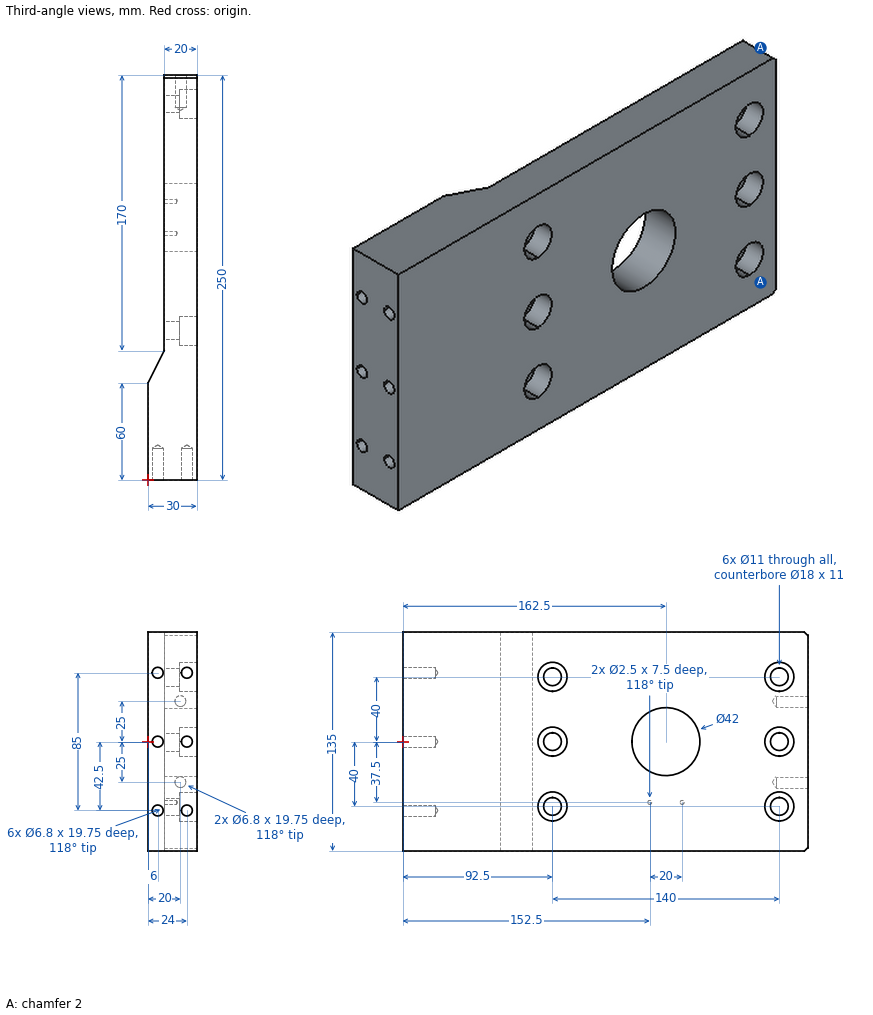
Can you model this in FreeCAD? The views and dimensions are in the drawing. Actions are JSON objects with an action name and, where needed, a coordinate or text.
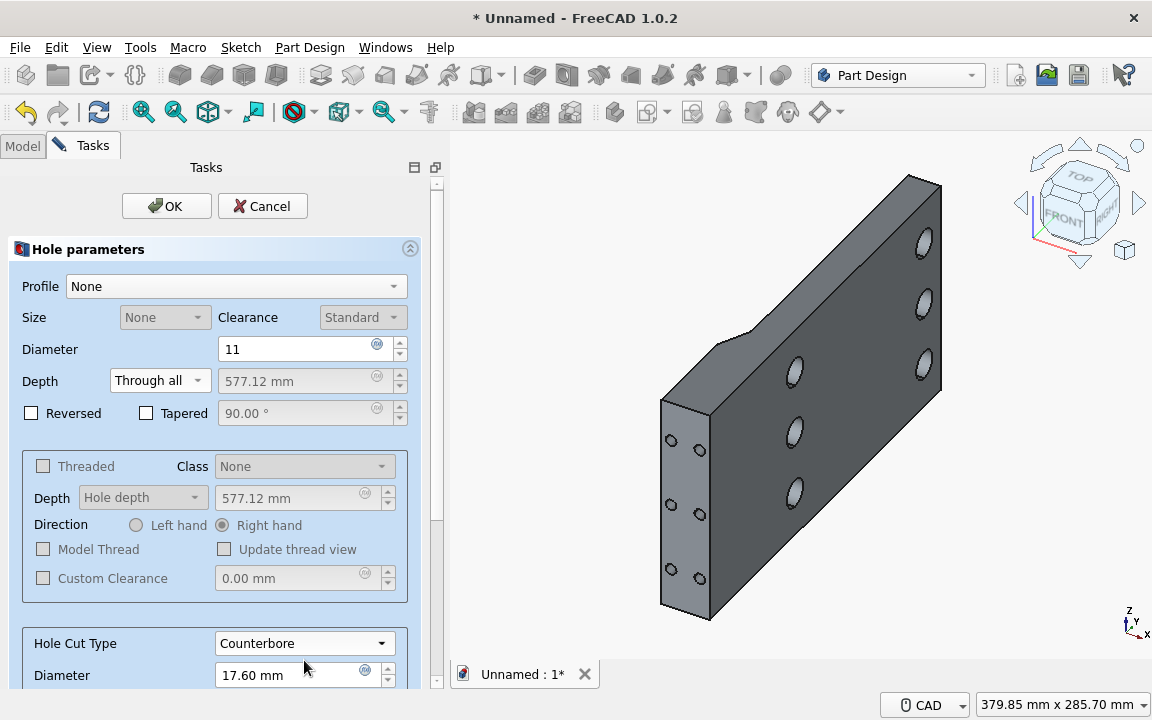
{"action": "triple_click", "coordinate": [298, 675]}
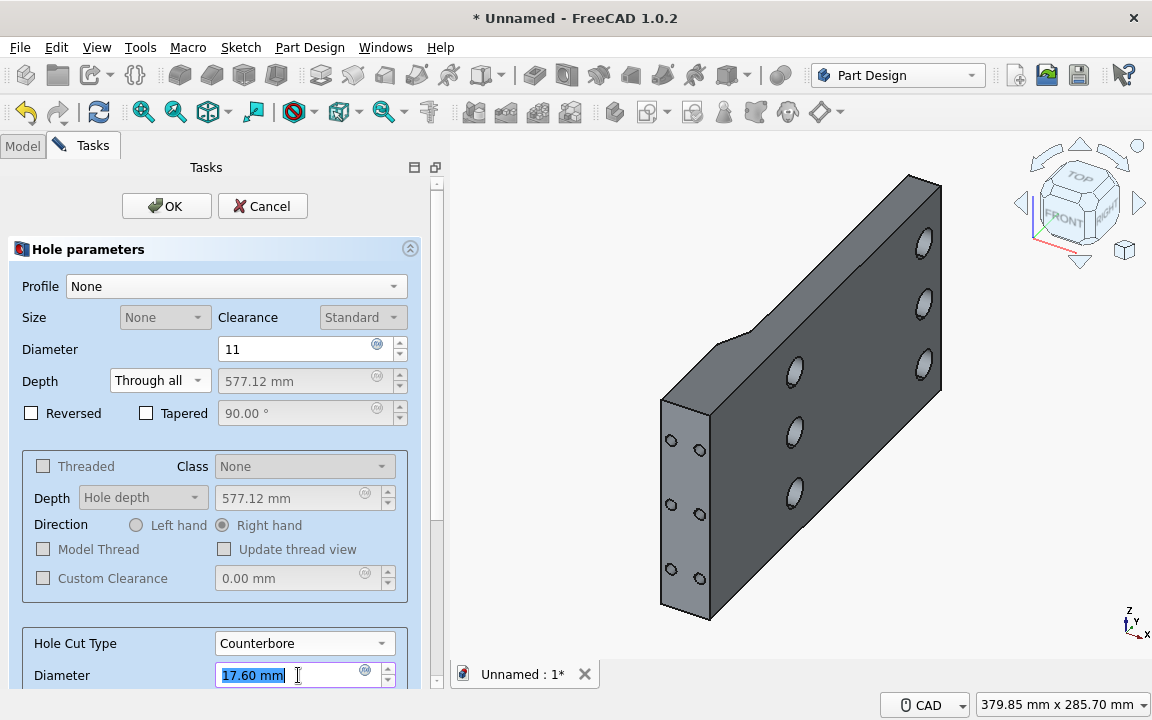
{"action": "type", "text": "18"}
{"action": "key", "text": "Tab"}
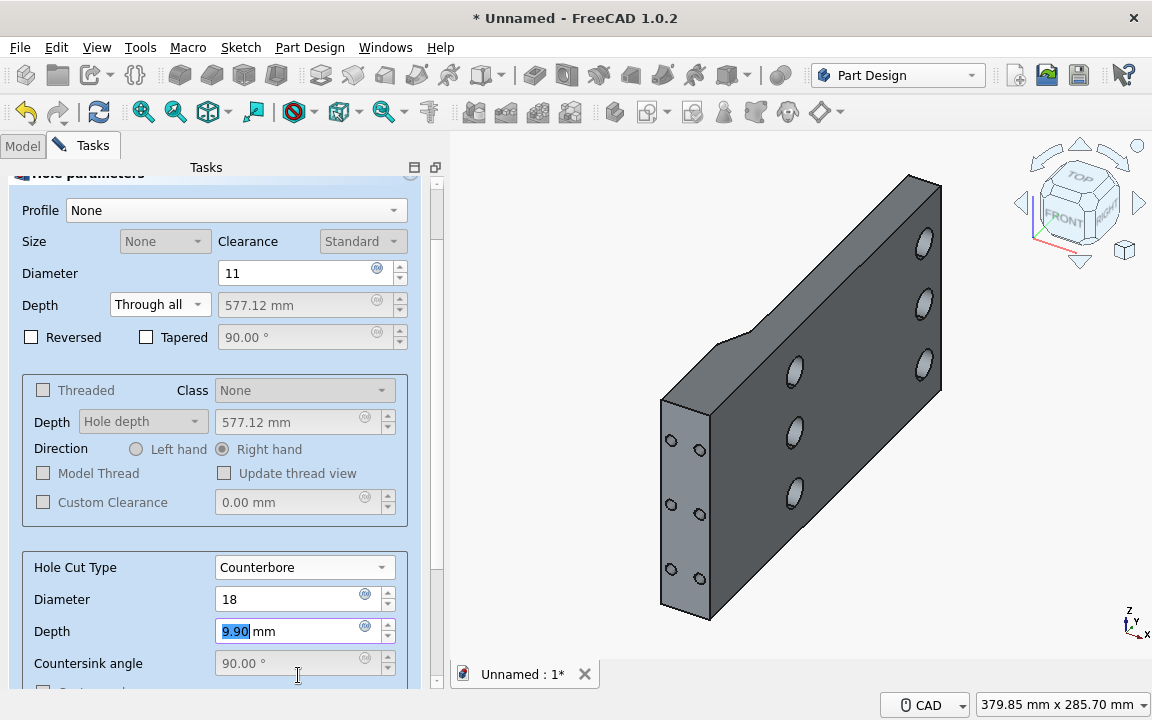
{"action": "type", "text": "11"}
{"action": "key", "text": "Tab"}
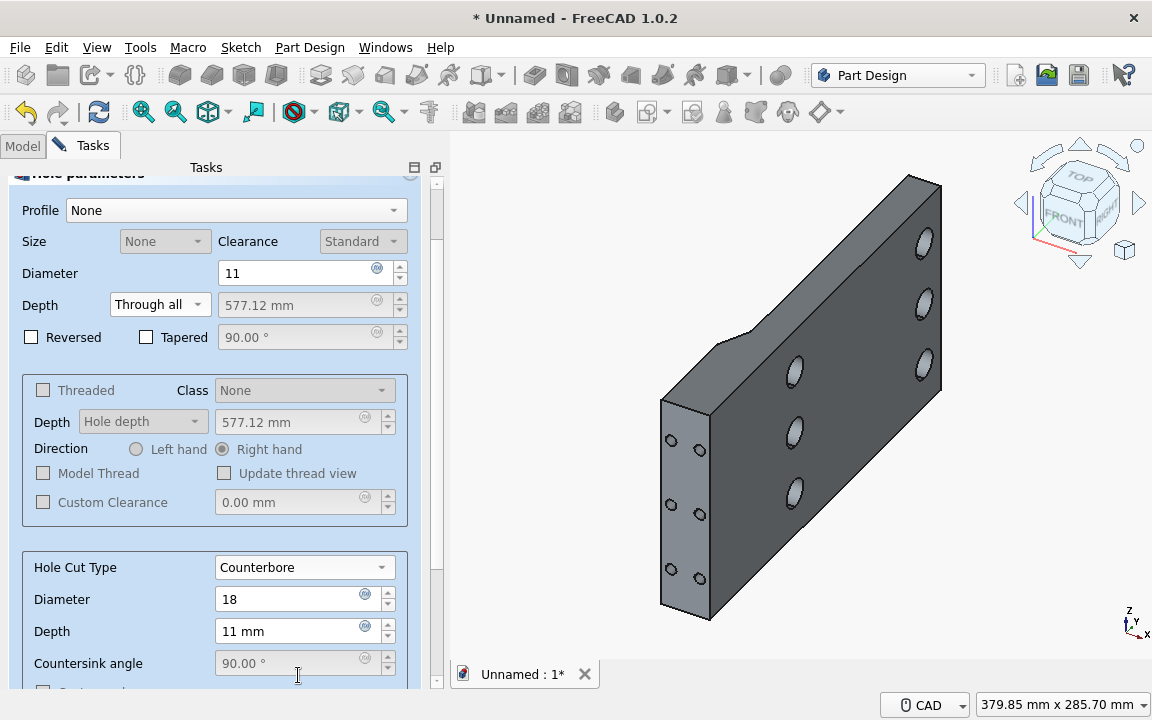
{"action": "scroll", "coordinate": [437, 432], "scroll_direction": "up", "scroll_amount": 3}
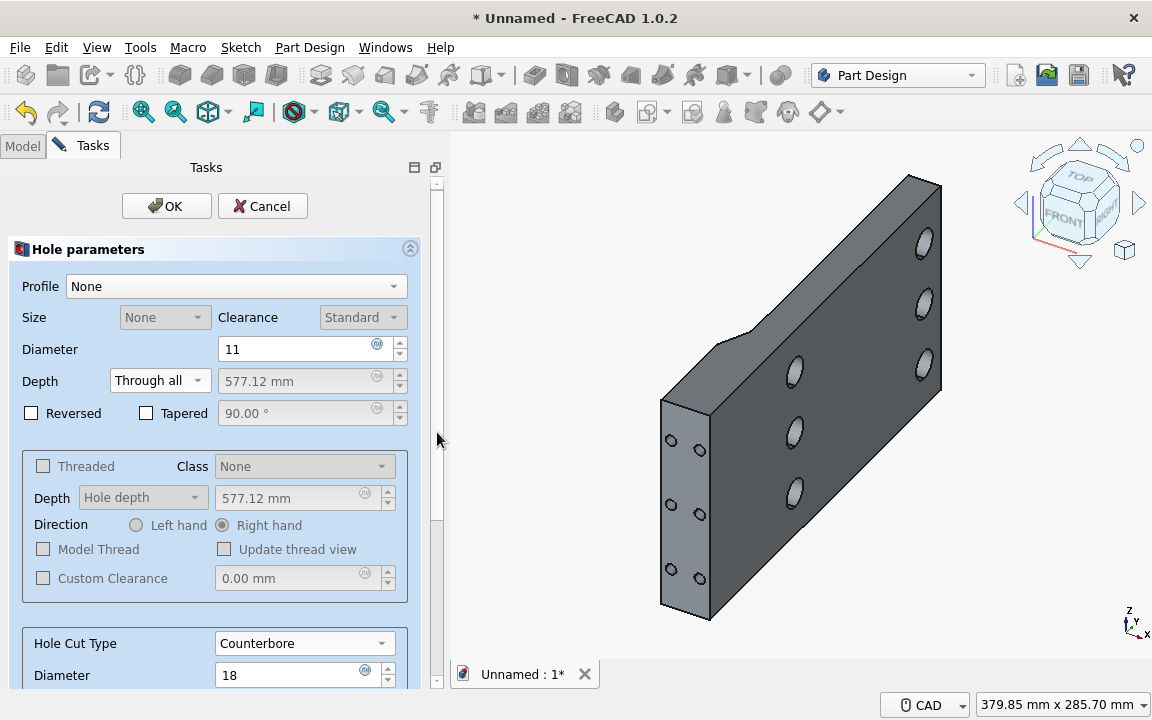
{"action": "left_click", "coordinate": [167, 206]}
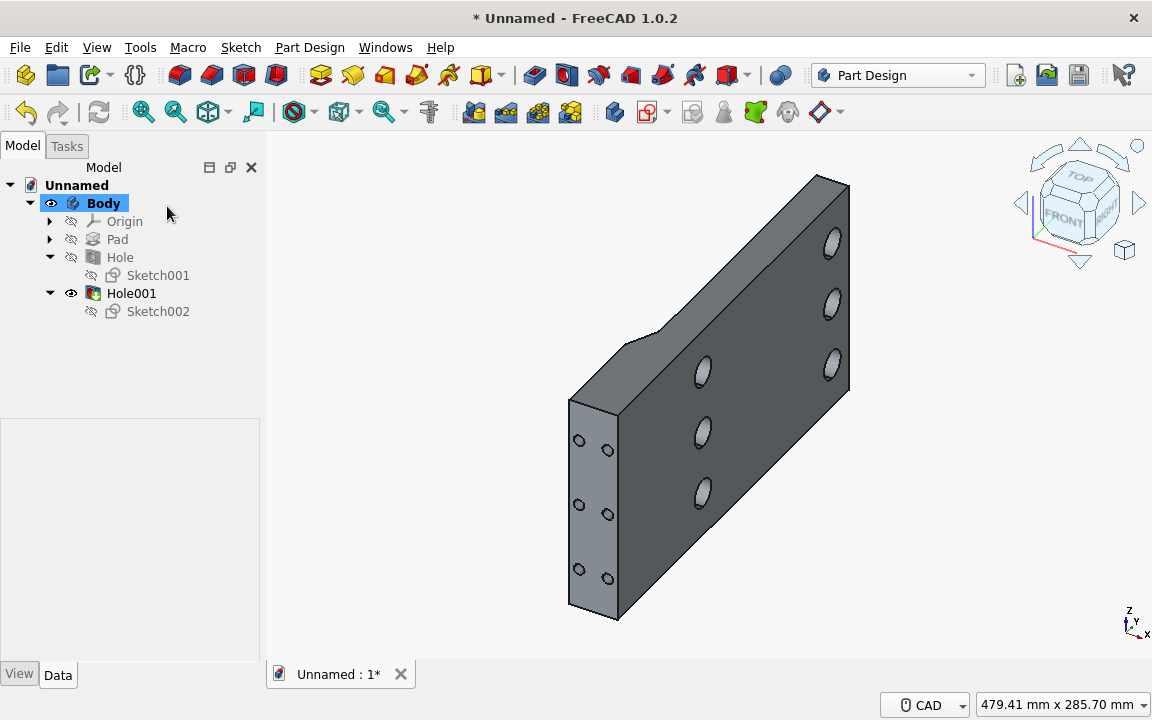
{"action": "key", "text": "6"}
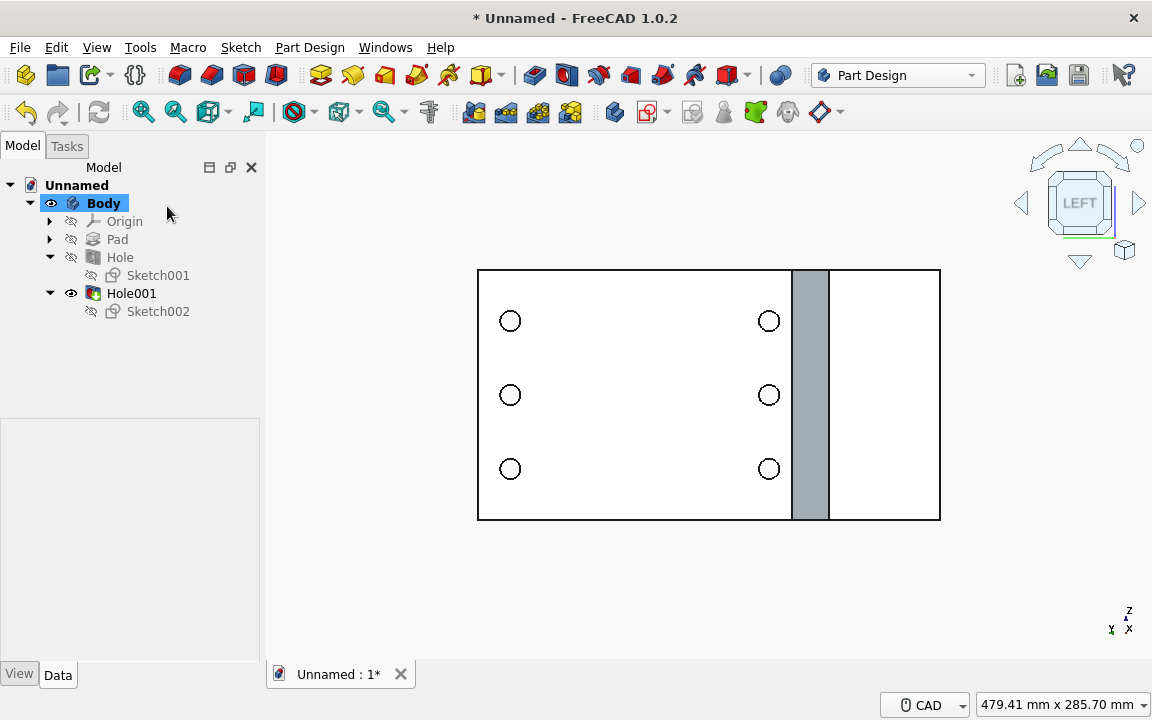
{"action": "left_click", "coordinate": [635, 394]}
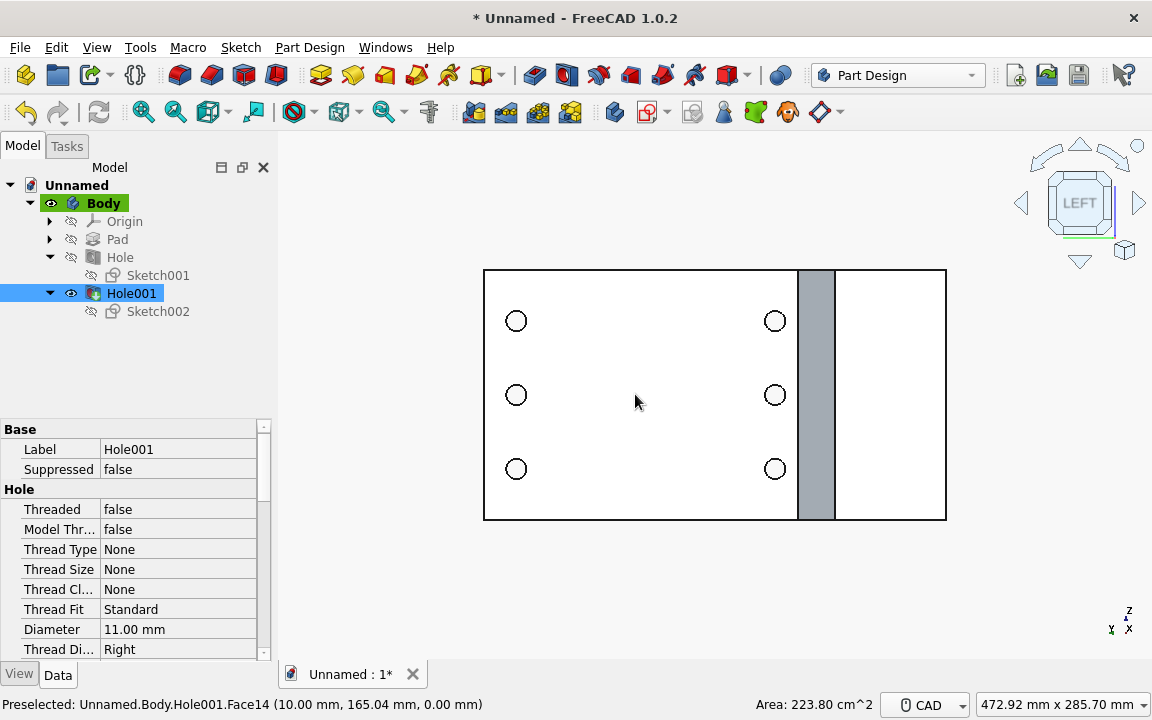
{"action": "left_click", "coordinate": [648, 112]}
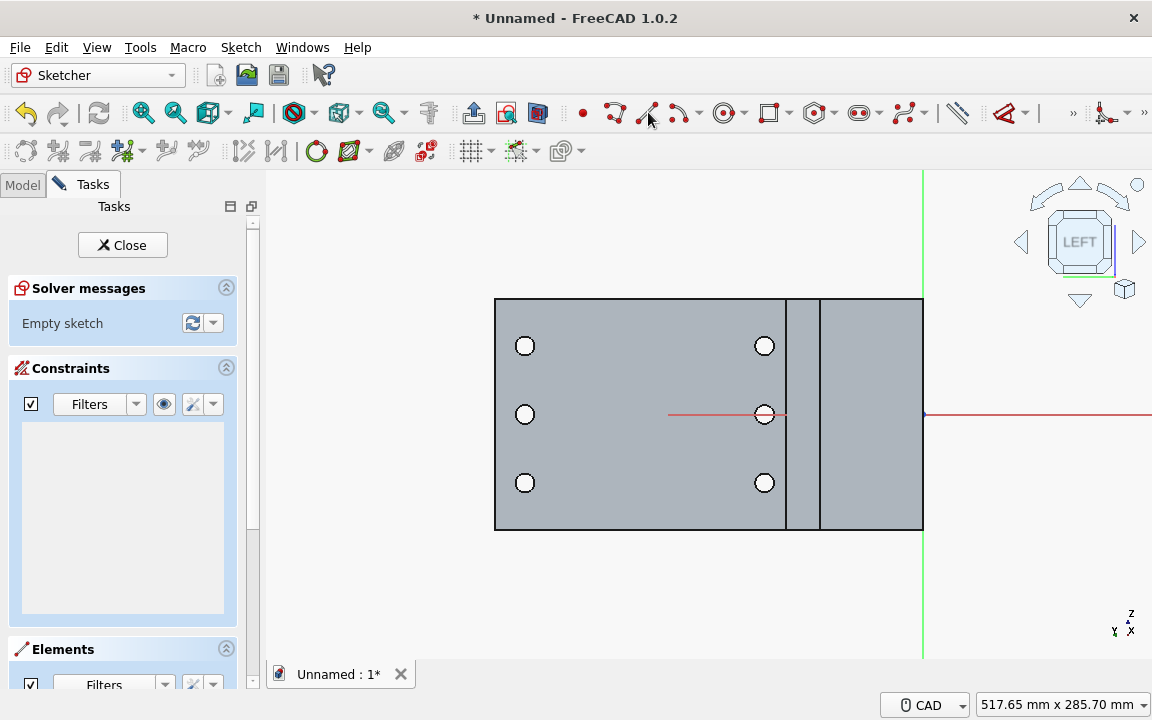
{"action": "scroll", "coordinate": [646, 415], "scroll_direction": "up", "scroll_amount": 7}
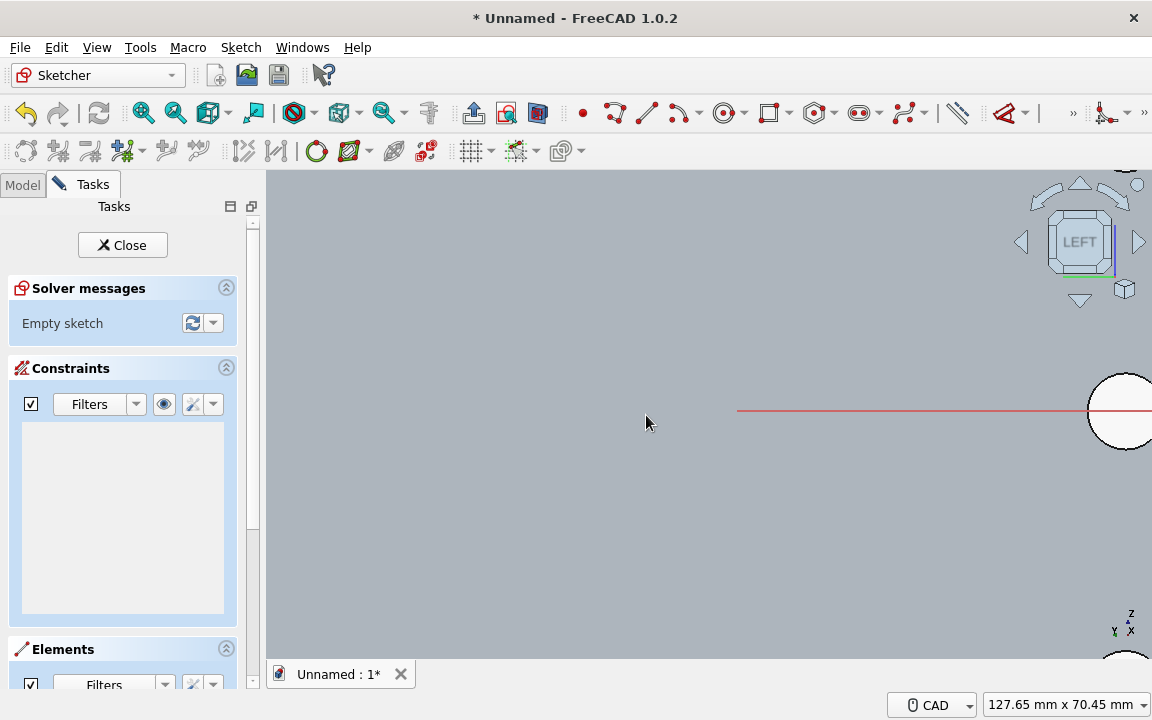
{"action": "left_click", "coordinate": [724, 114]}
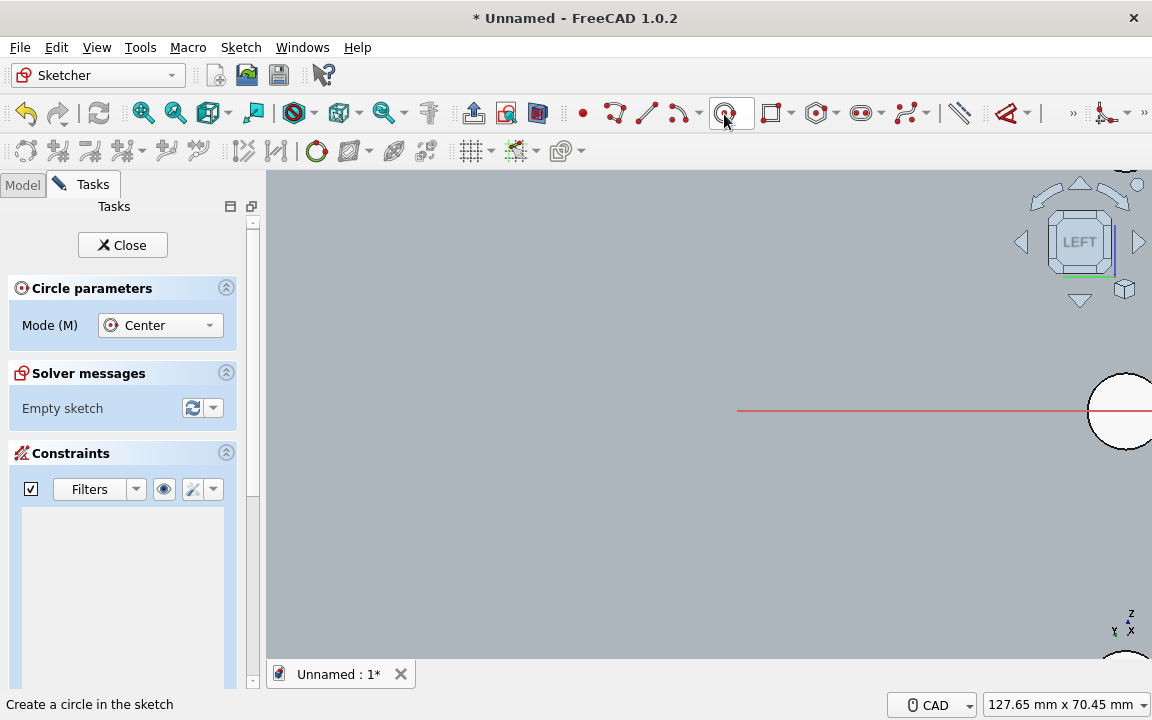
{"action": "left_click", "coordinate": [640, 411]}
{"action": "mouse_move", "coordinate": [743, 308]}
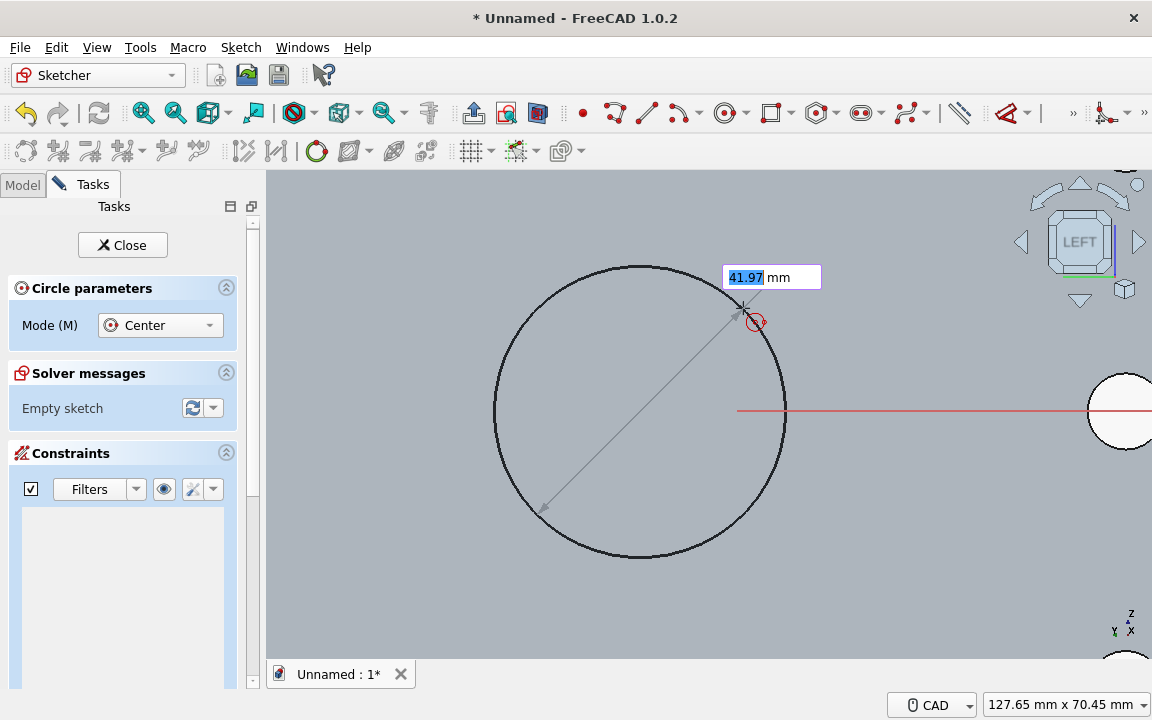
{"action": "type", "text": "42"}
{"action": "key", "text": "Return"}
{"action": "key", "text": "Escape"}